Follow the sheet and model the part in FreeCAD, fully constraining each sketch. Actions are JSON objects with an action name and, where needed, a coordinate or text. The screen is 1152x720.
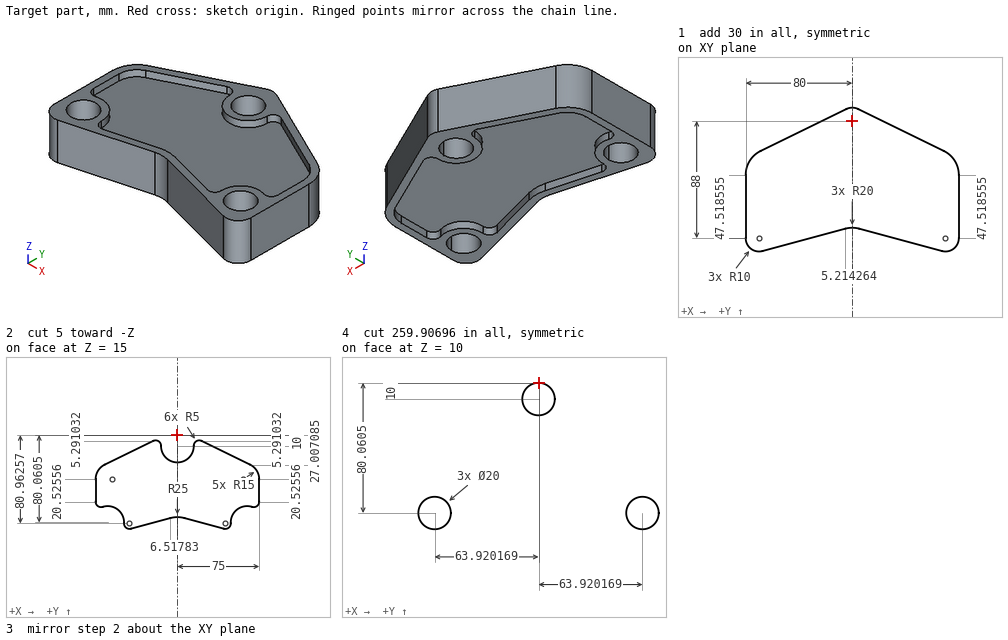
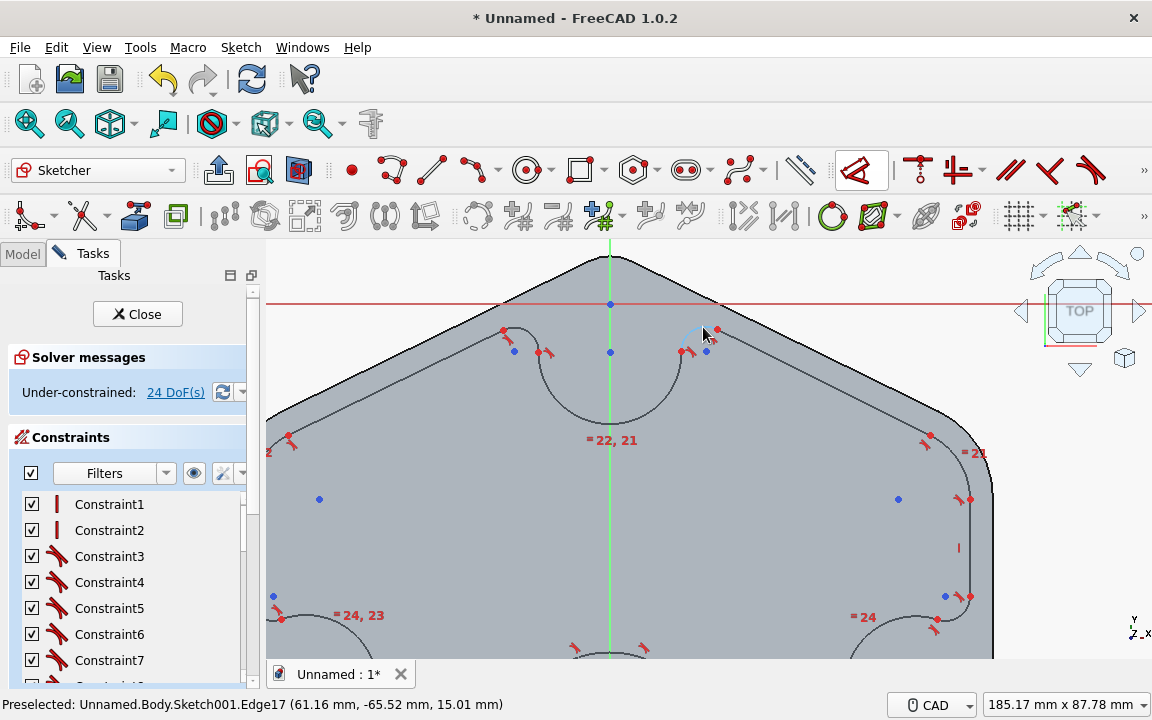
{"action": "left_click", "coordinate": [702, 327]}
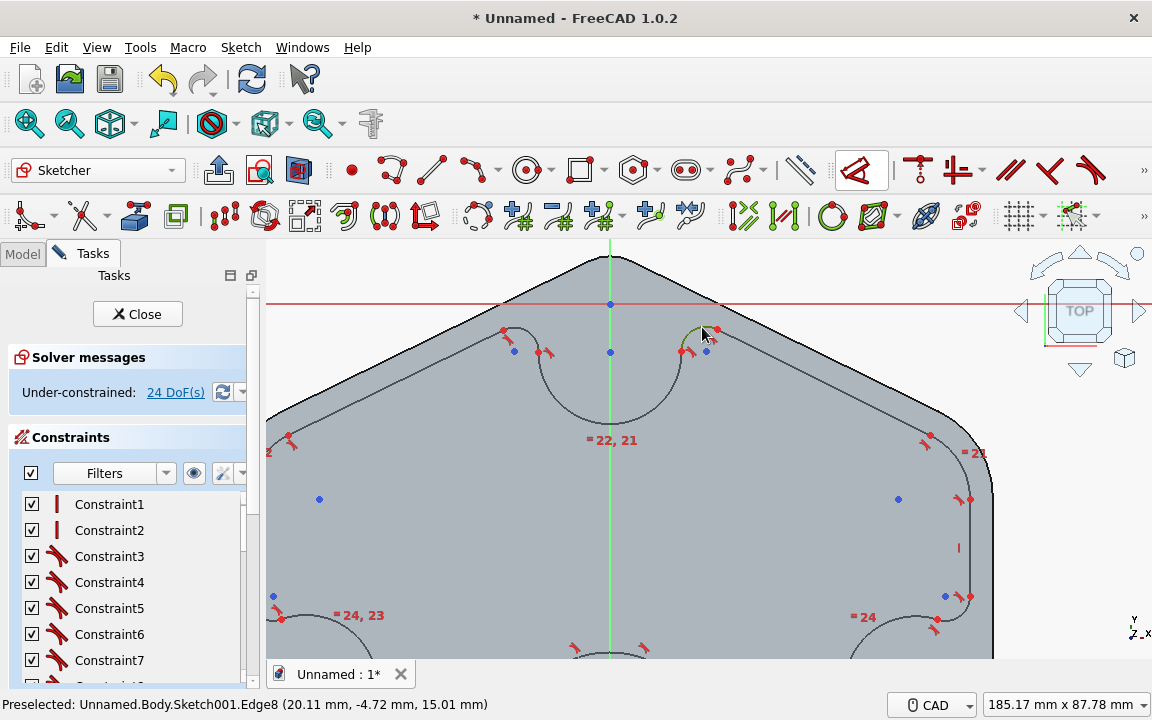
{"action": "left_click", "coordinate": [534, 338]}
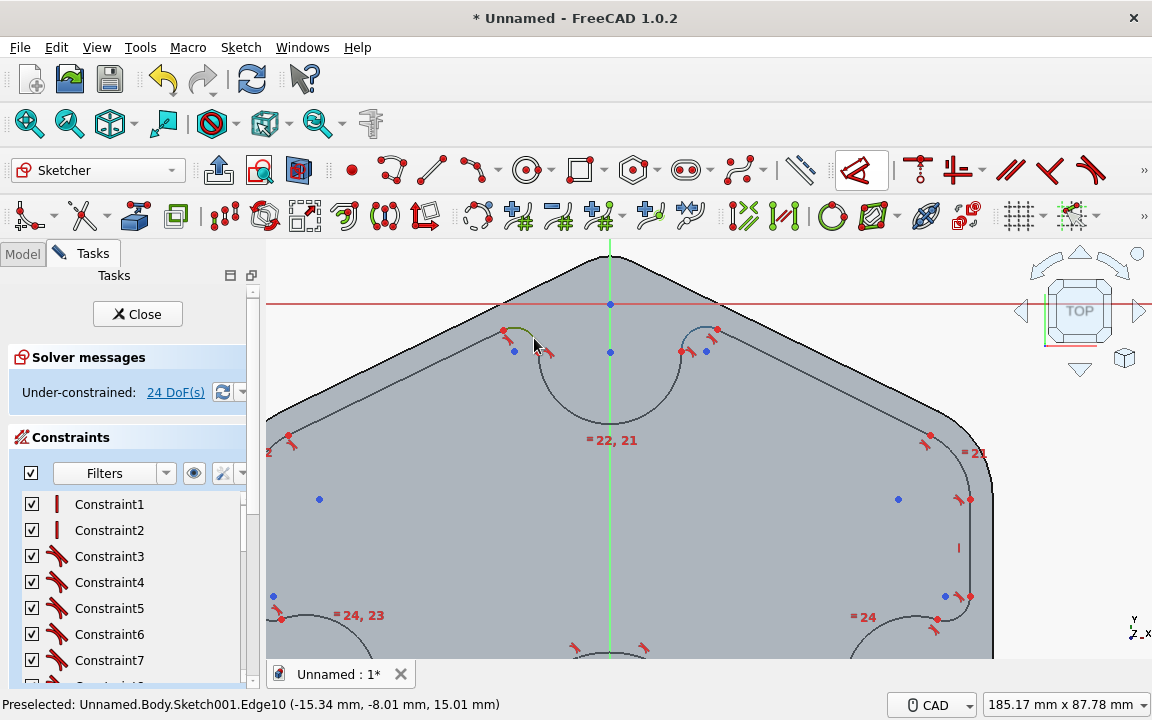
{"action": "scroll", "coordinate": [702, 326], "scroll_direction": "down", "scroll_amount": 2}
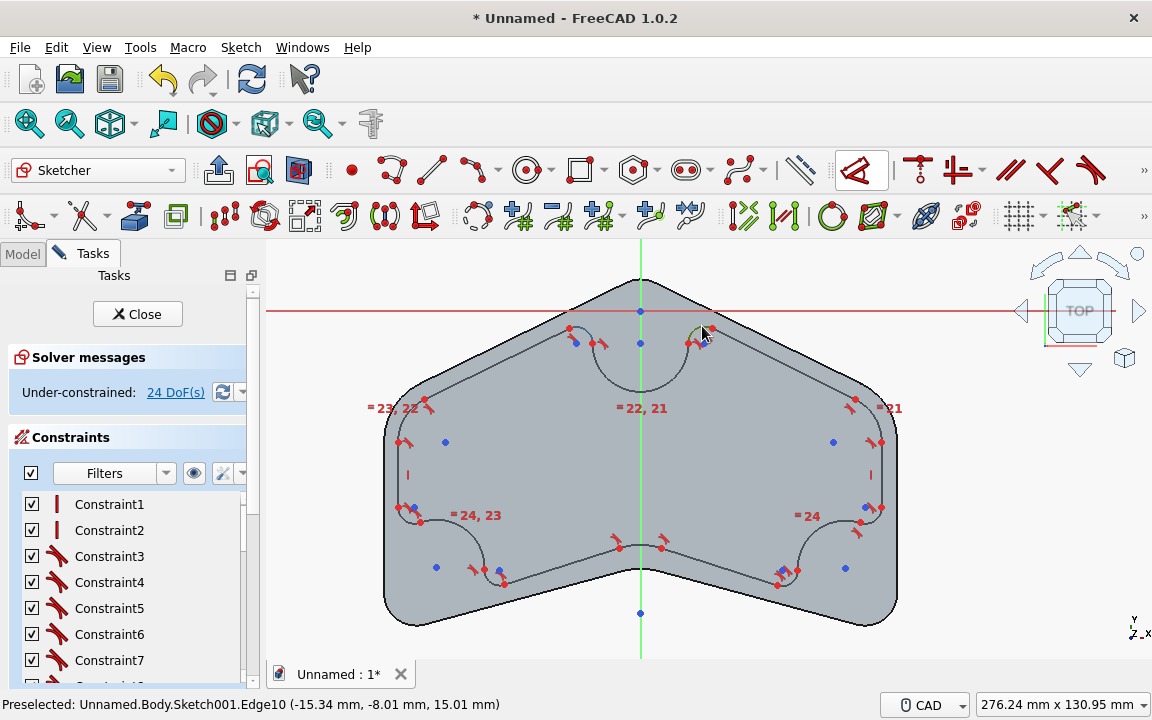
{"action": "scroll", "coordinate": [401, 516], "scroll_direction": "up", "scroll_amount": 2}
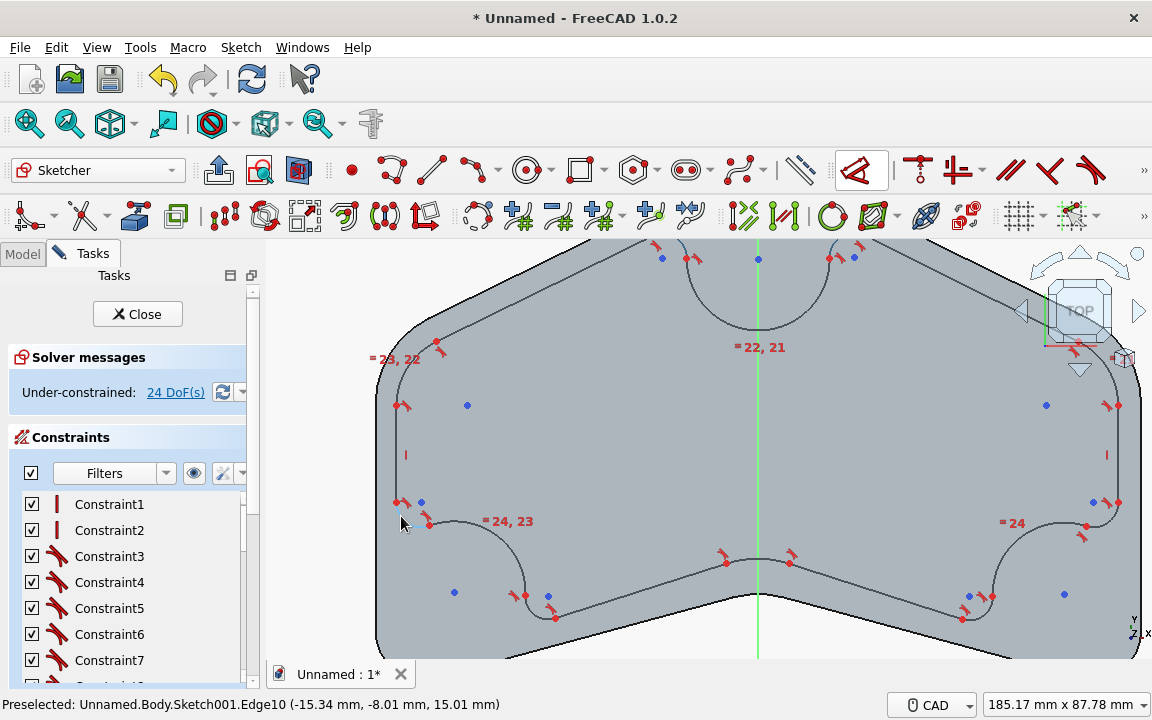
{"action": "left_click", "coordinate": [400, 516]}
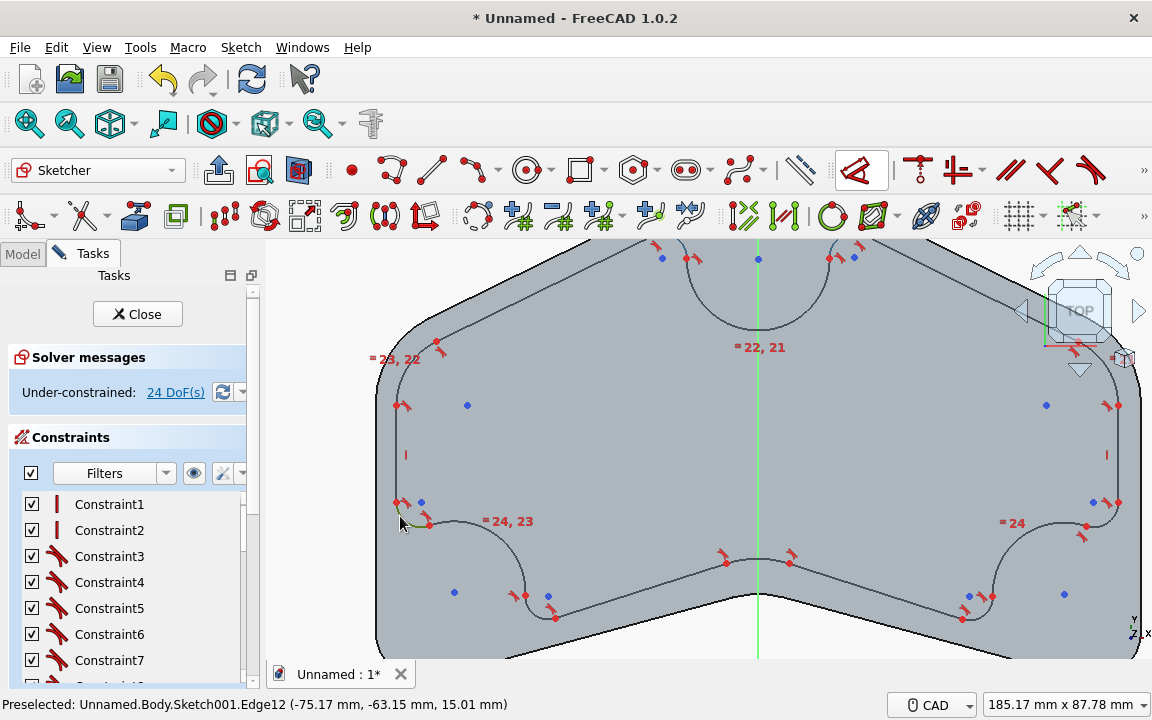
{"action": "left_click", "coordinate": [529, 608]}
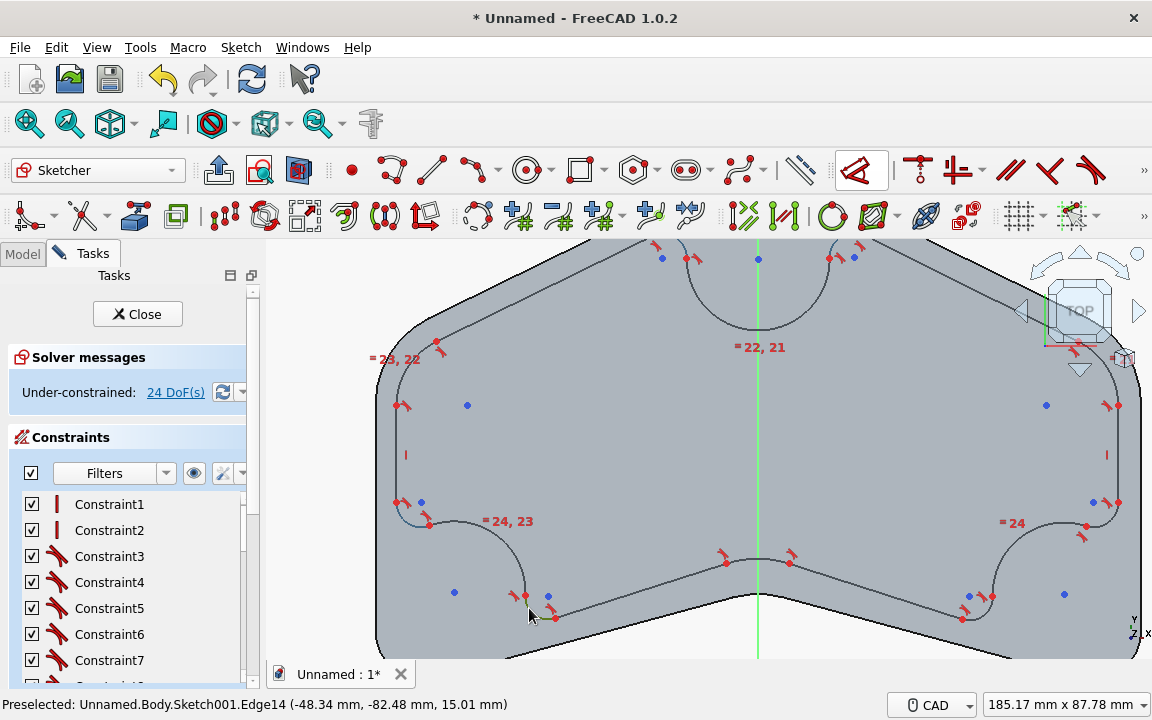
{"action": "left_click", "coordinate": [975, 620]}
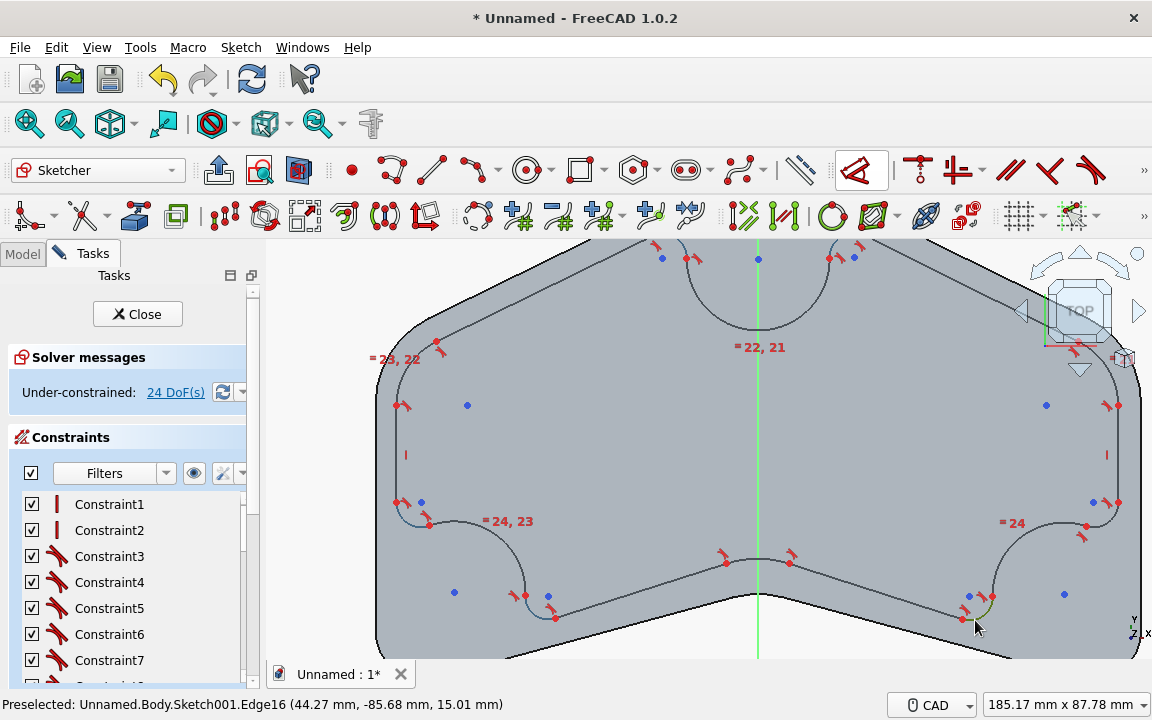
{"action": "scroll", "coordinate": [401, 517], "scroll_direction": "down", "scroll_amount": 2}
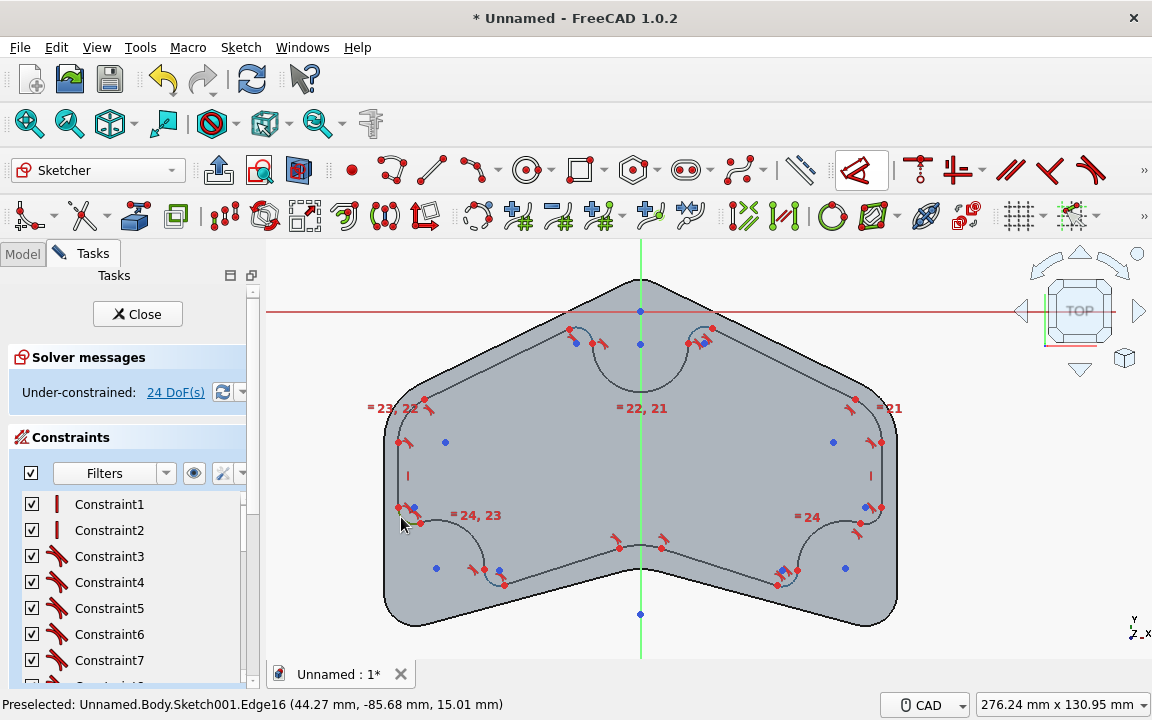
{"action": "scroll", "coordinate": [869, 524], "scroll_direction": "up", "scroll_amount": 3}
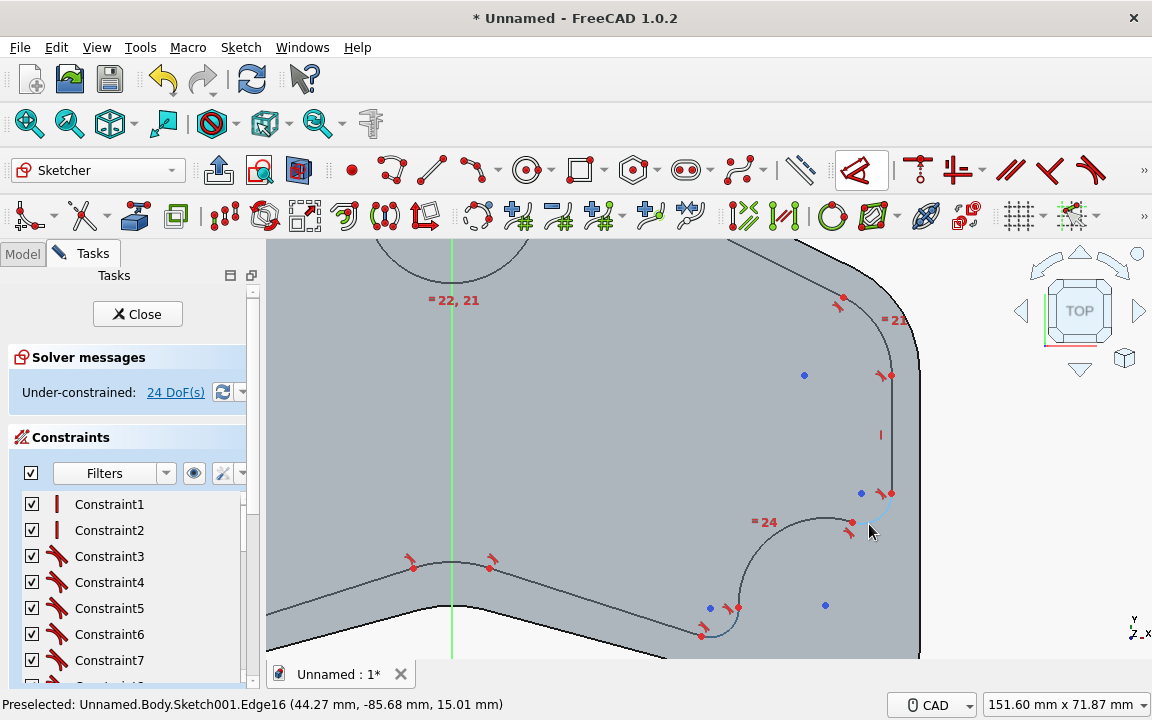
{"action": "left_click", "coordinate": [869, 523]}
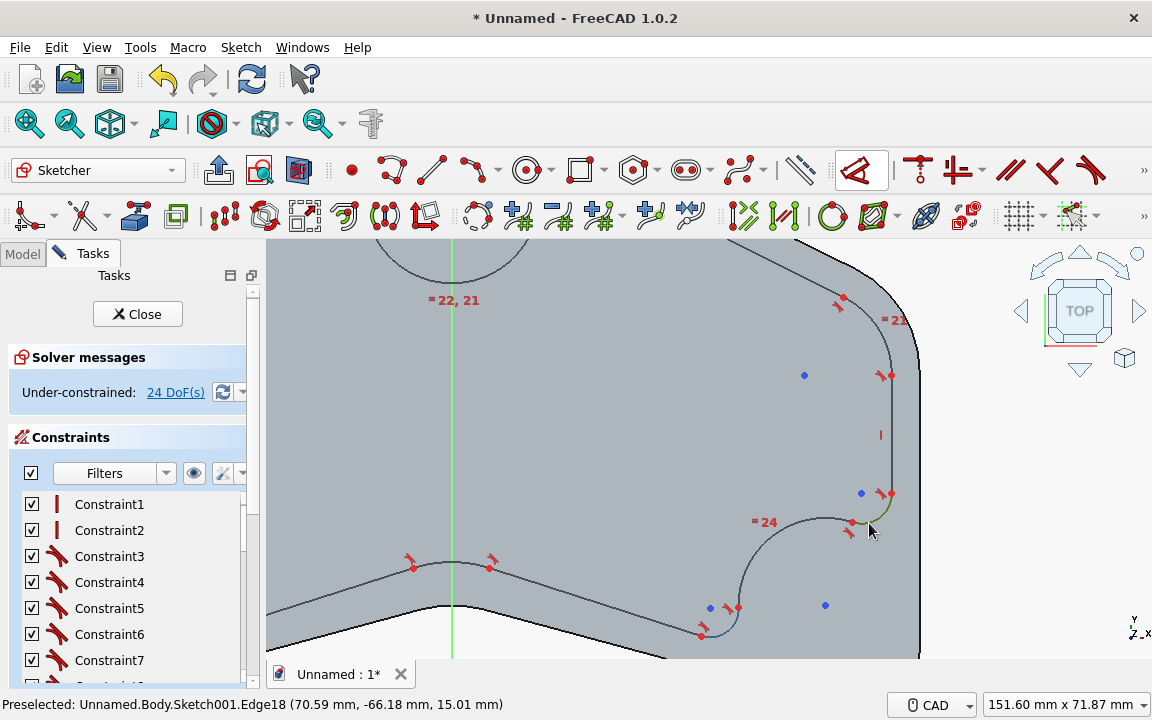
{"action": "key", "text": "e"}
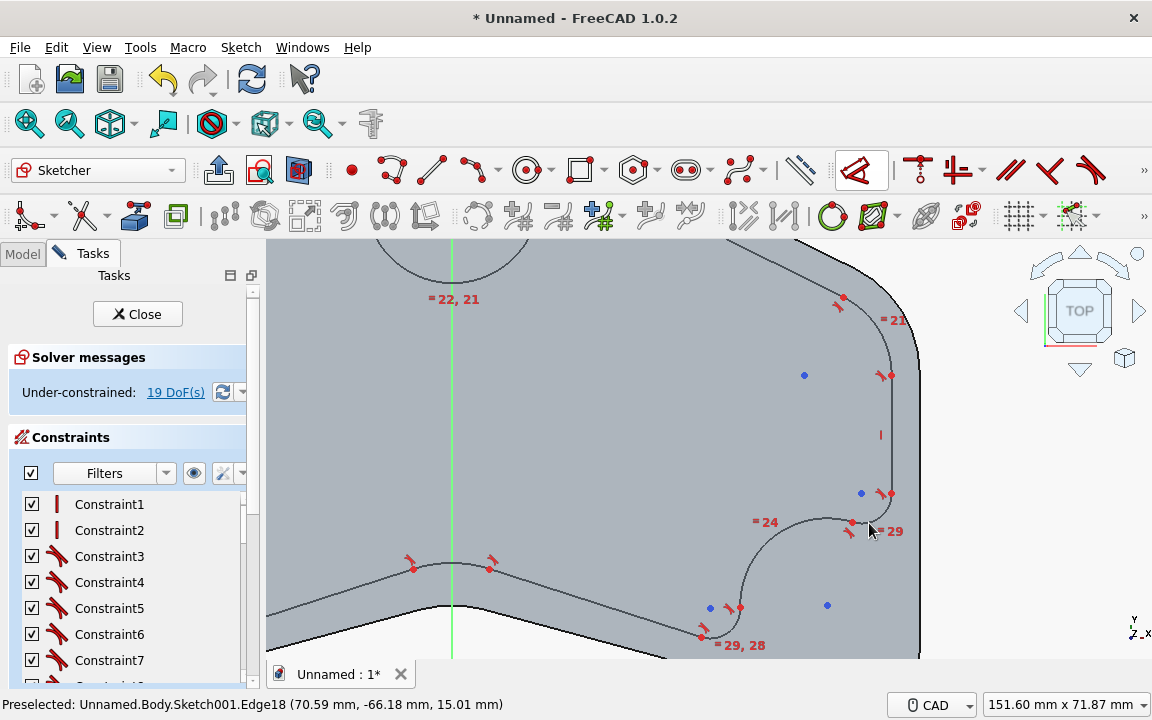
{"action": "scroll", "coordinate": [869, 524], "scroll_direction": "down", "scroll_amount": 3}